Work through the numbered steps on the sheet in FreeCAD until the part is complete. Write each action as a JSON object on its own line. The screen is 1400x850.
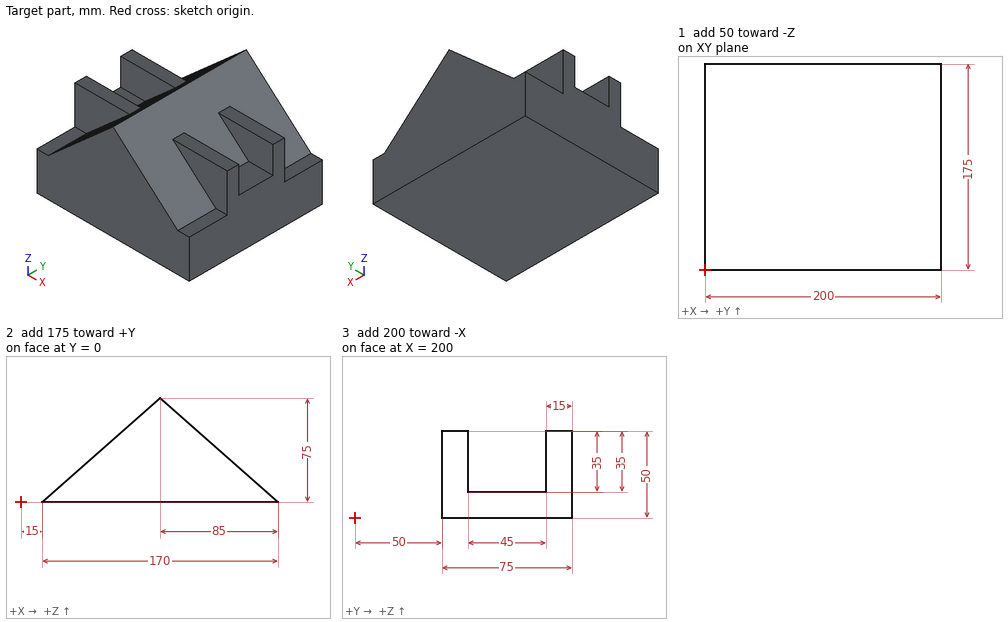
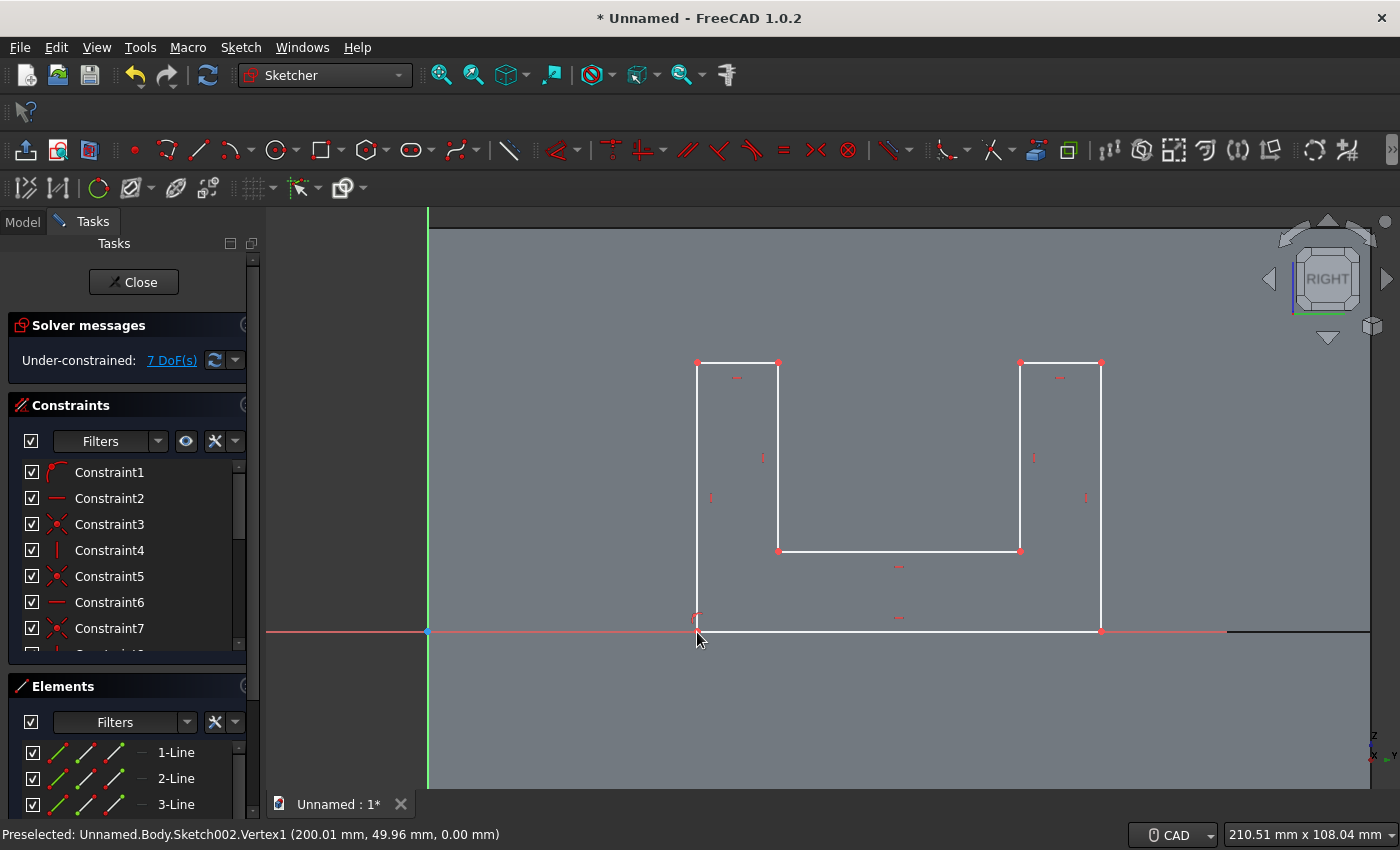
{"action": "left_click", "coordinate": [556, 150]}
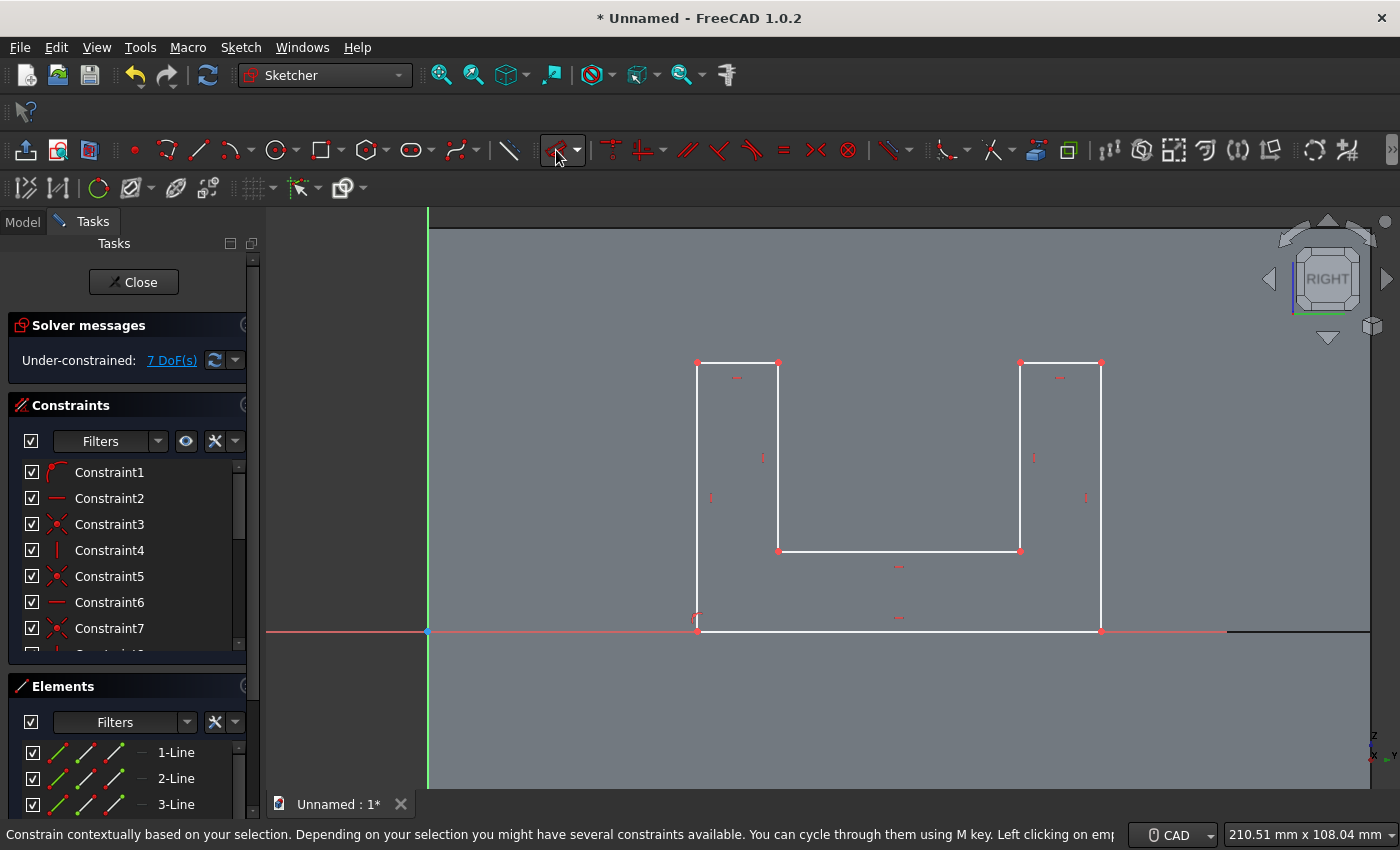
{"action": "left_click", "coordinate": [818, 632]}
{"action": "left_click", "coordinate": [899, 666]}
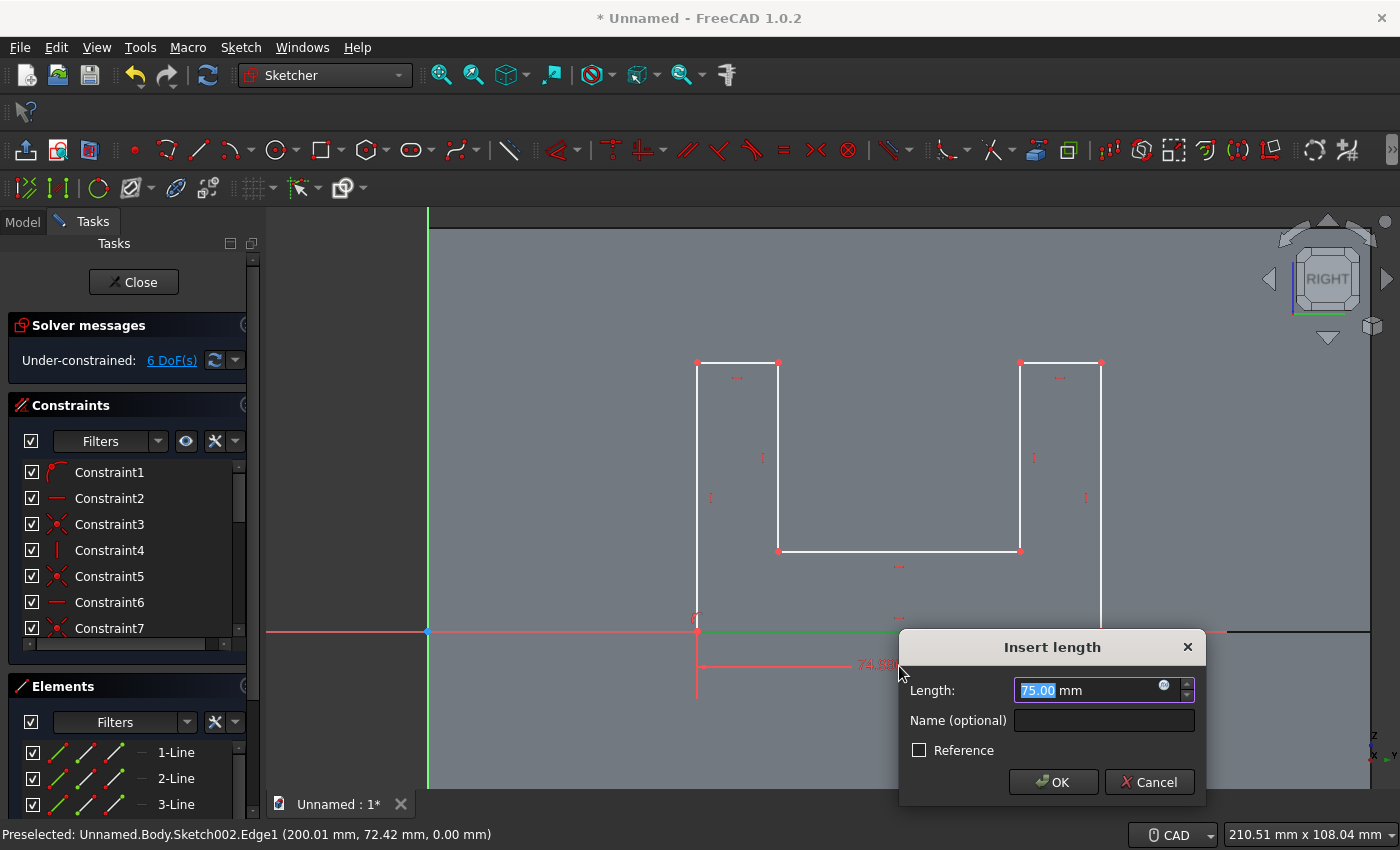
{"action": "type", "text": "75"}
{"action": "key", "text": "Return"}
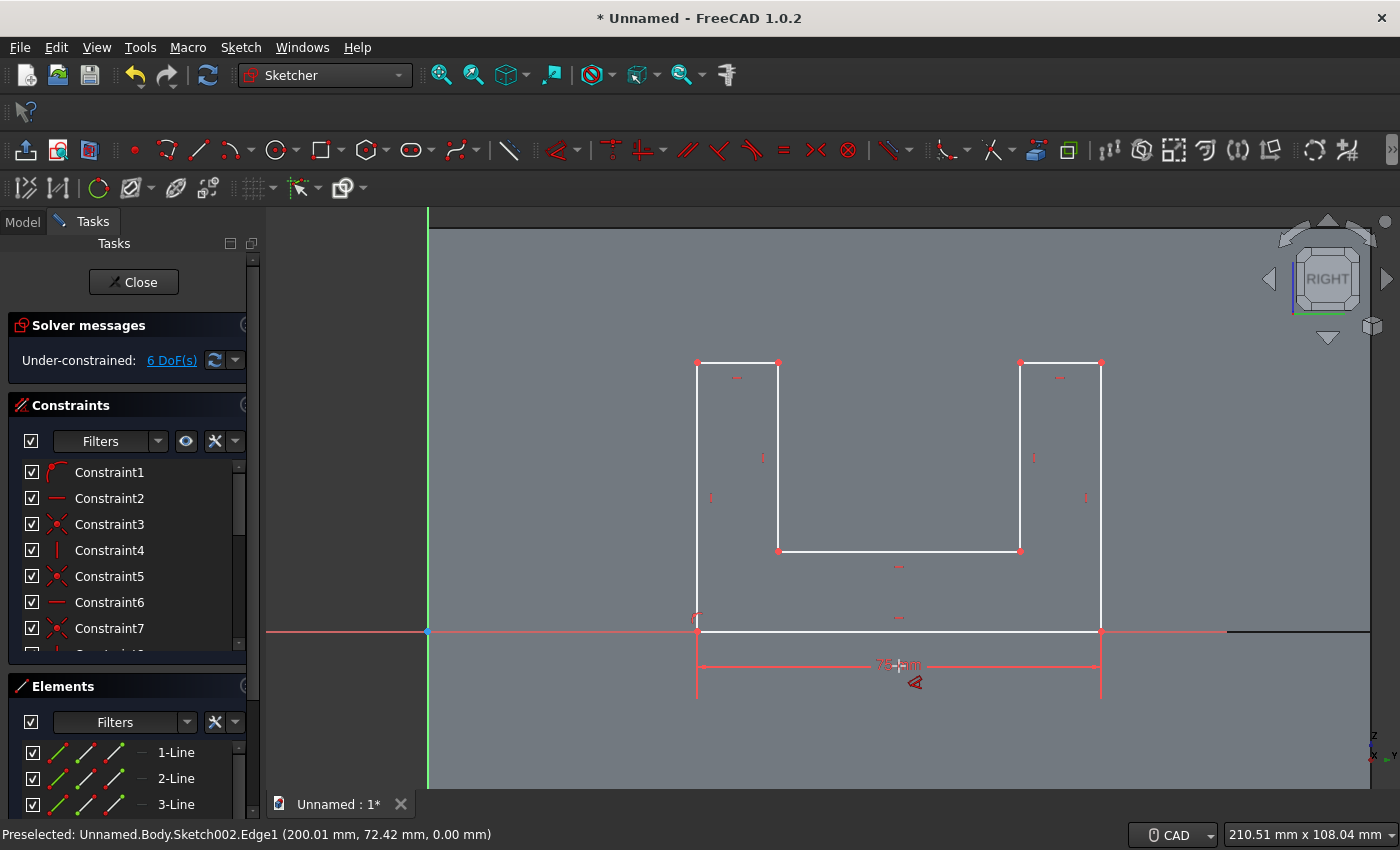
{"action": "left_click", "coordinate": [1101, 551]}
{"action": "left_click", "coordinate": [1135, 497]}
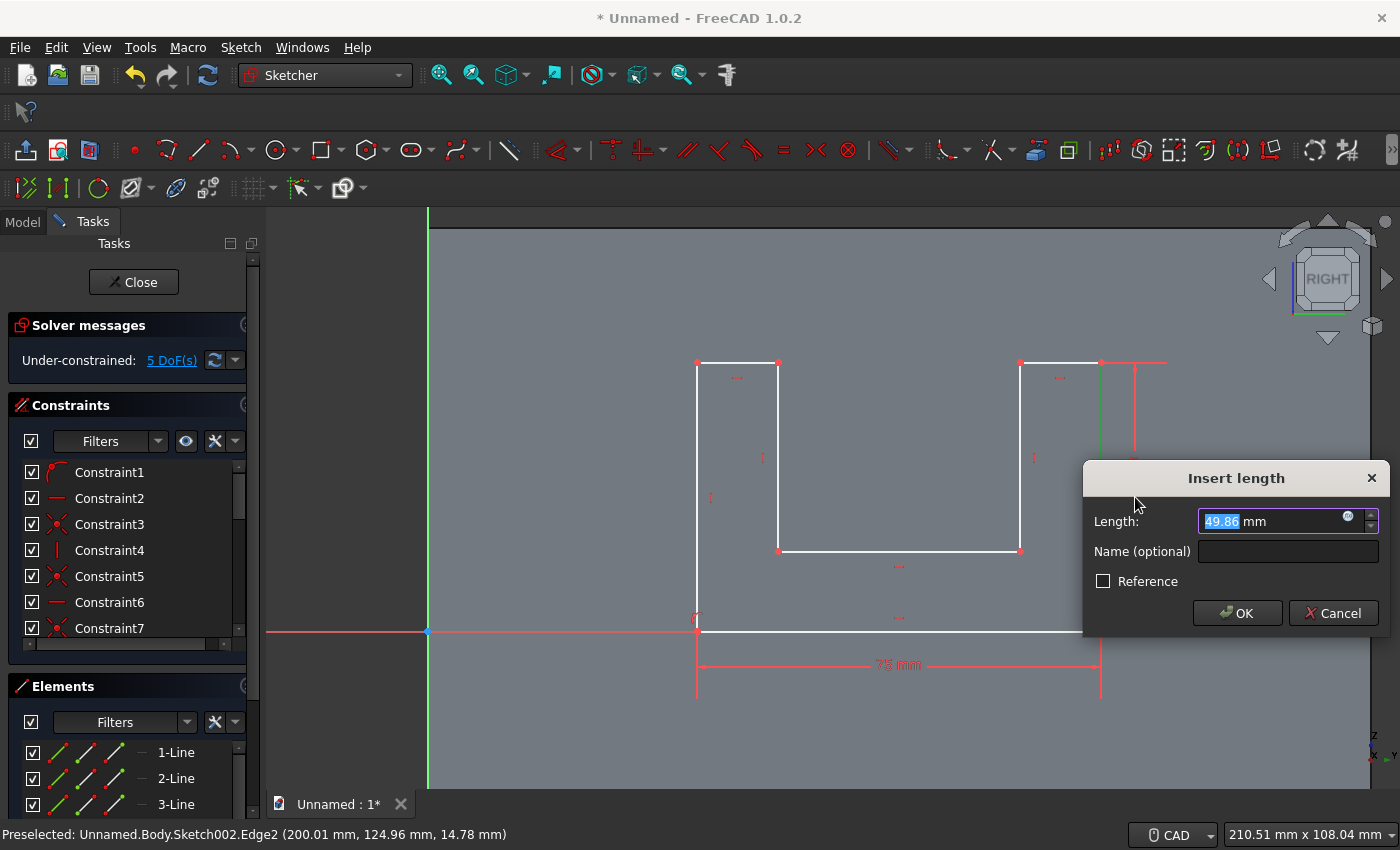
{"action": "type", "text": "50"}
{"action": "key", "text": "Return"}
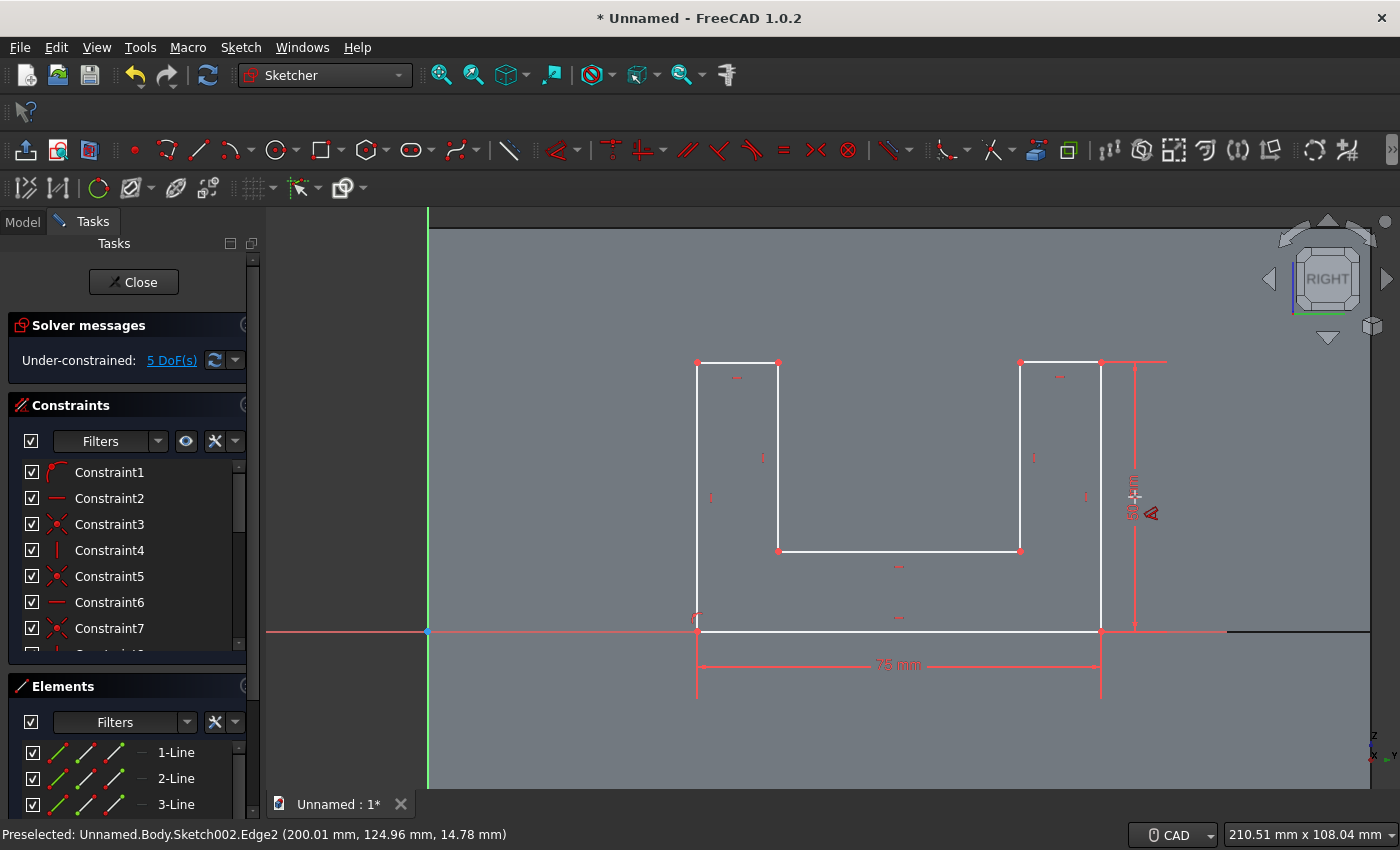
{"action": "left_click", "coordinate": [1077, 362]}
{"action": "left_click", "coordinate": [1061, 328]}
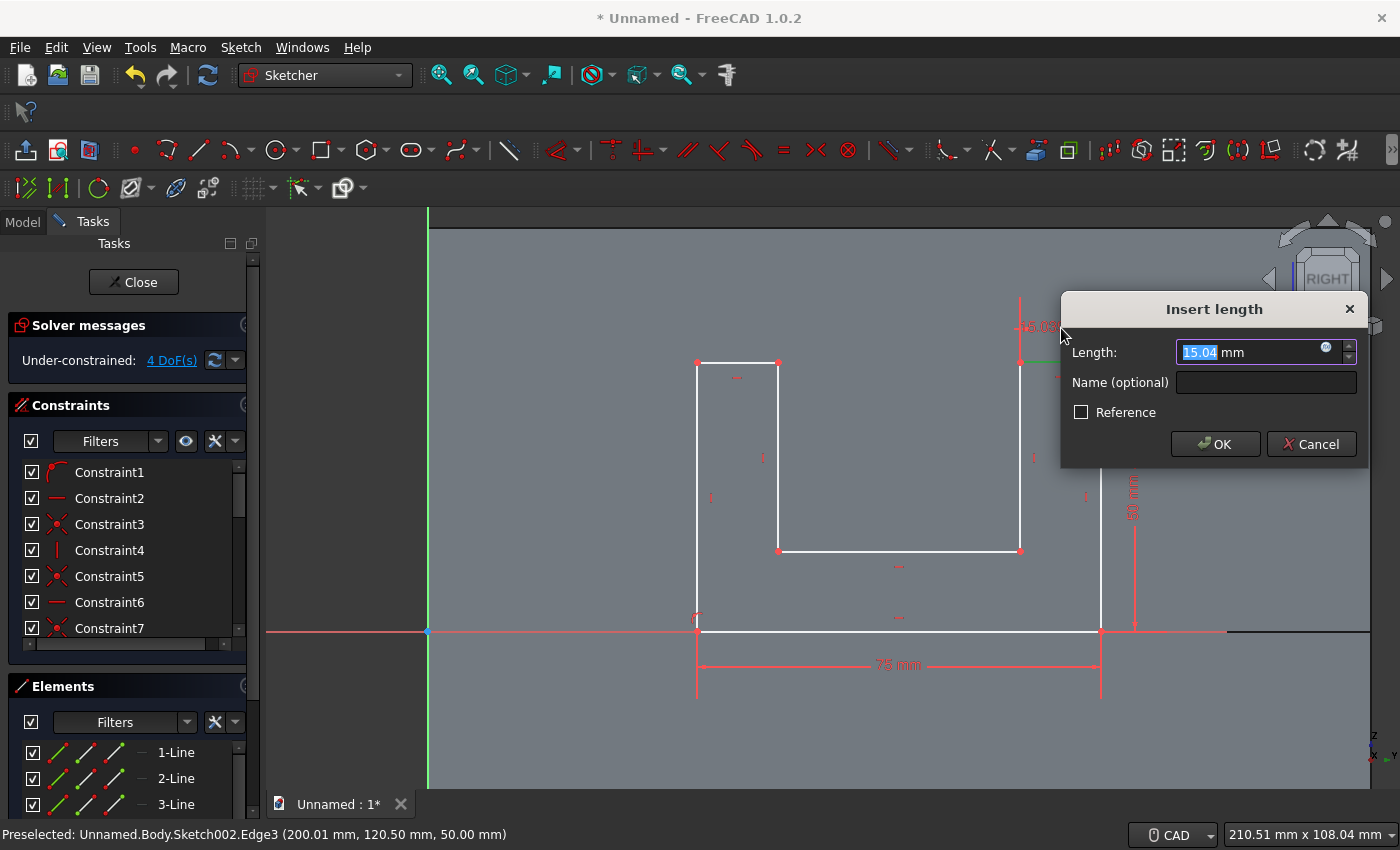
{"action": "type", "text": "15"}
{"action": "key", "text": "Return"}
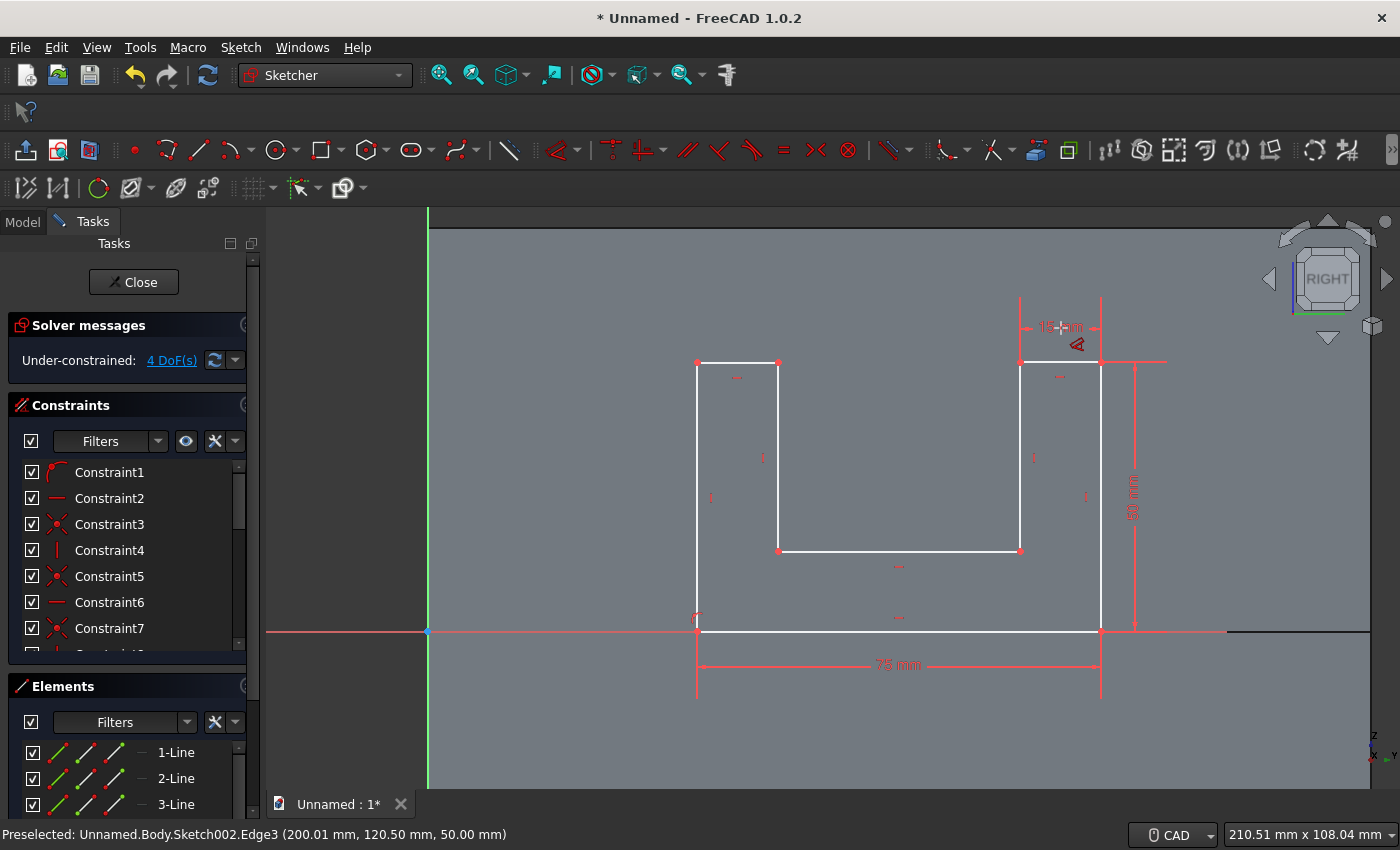
{"action": "left_click", "coordinate": [1020, 419]}
{"action": "left_click", "coordinate": [1054, 457]}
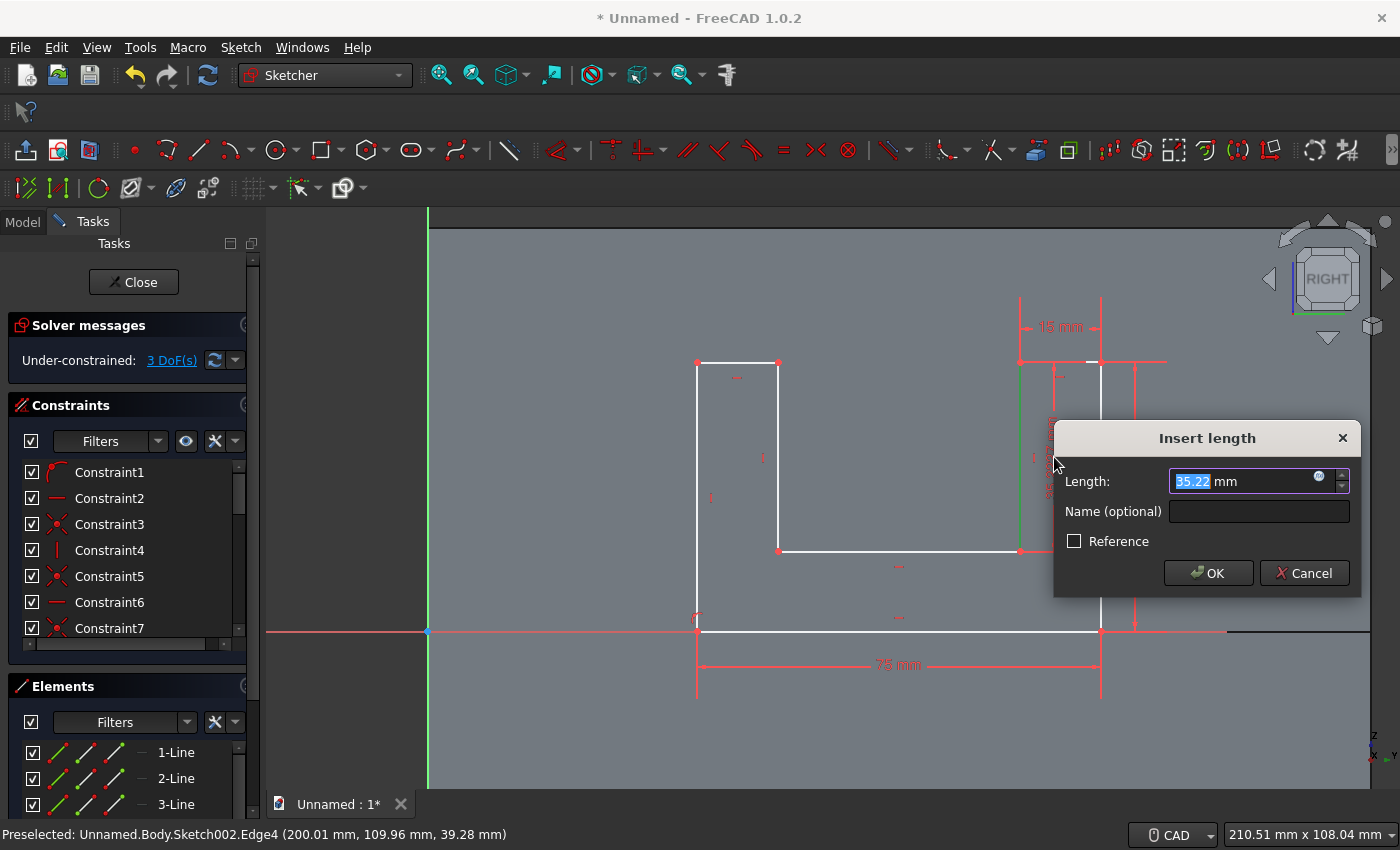
{"action": "type", "text": "35"}
{"action": "key", "text": "Return"}